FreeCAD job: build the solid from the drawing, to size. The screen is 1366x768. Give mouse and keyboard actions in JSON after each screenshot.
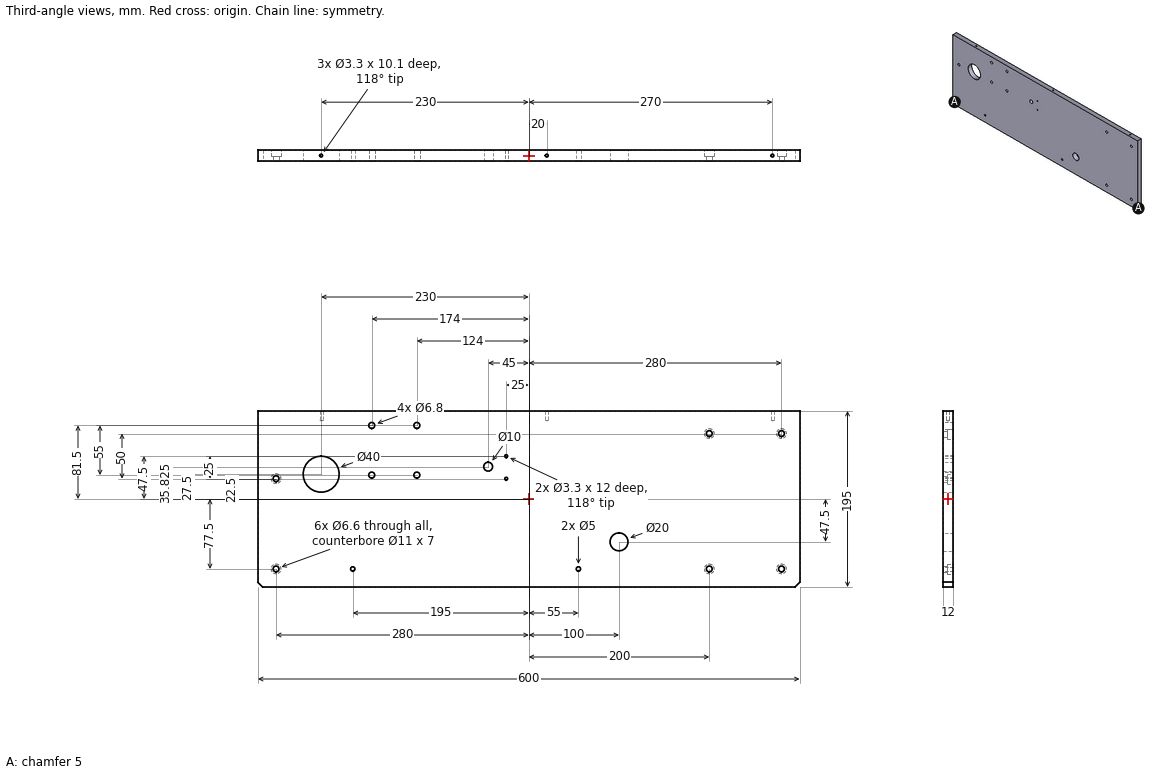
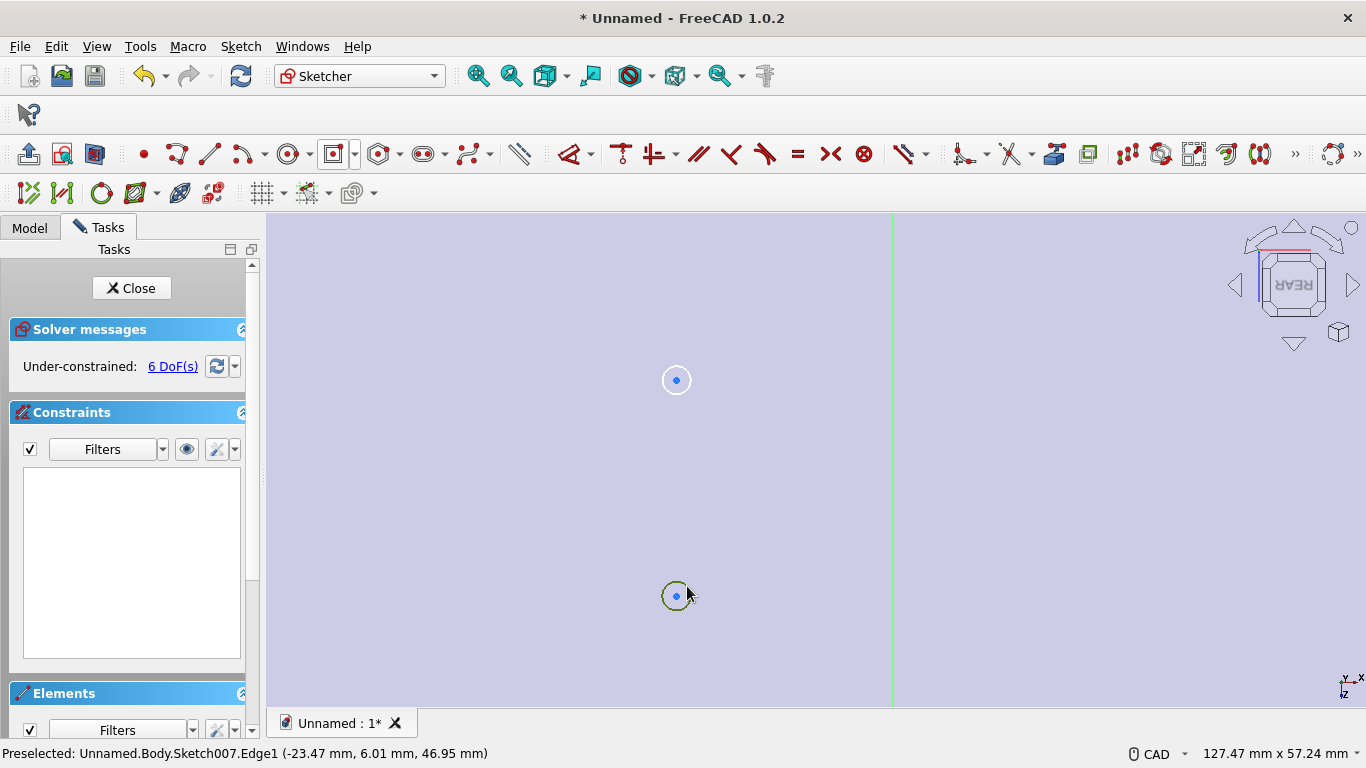
{"action": "left_click", "coordinate": [687, 370]}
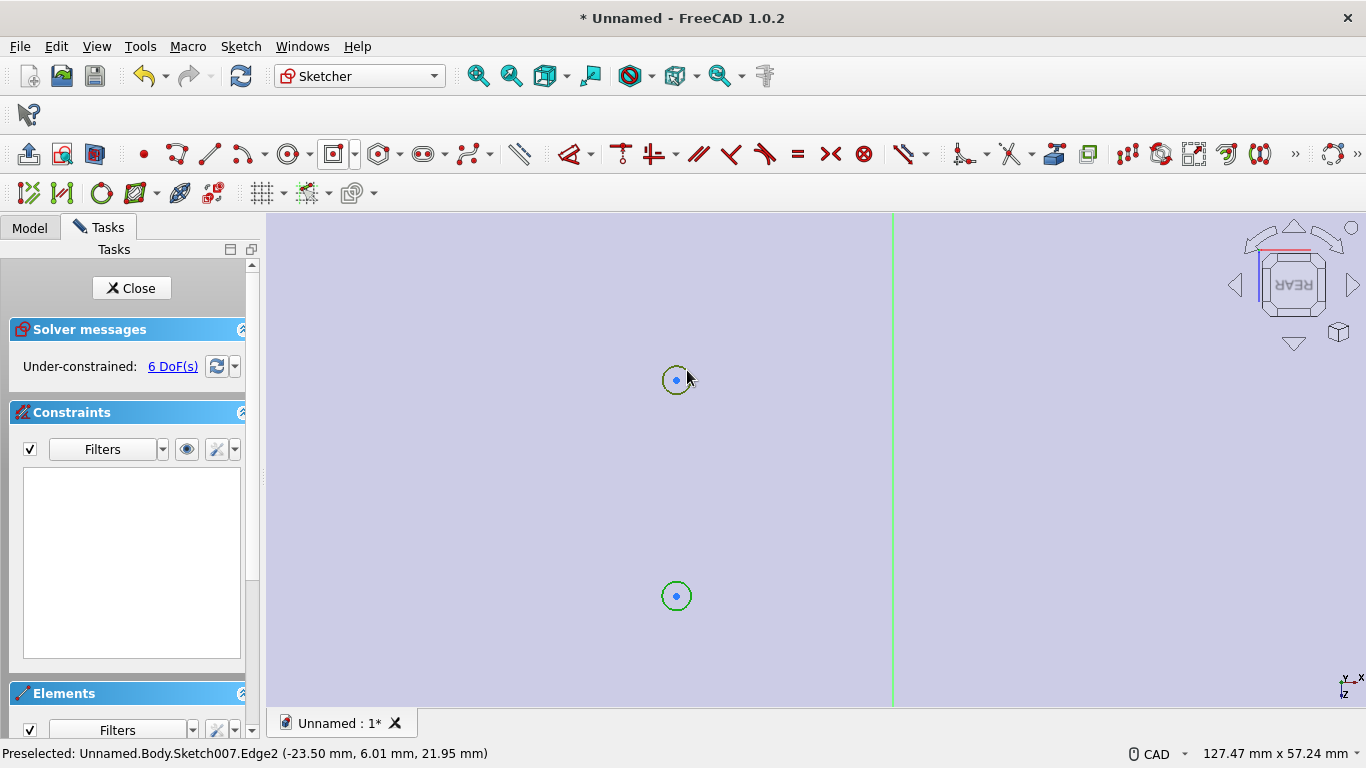
{"action": "left_click", "coordinate": [798, 154]}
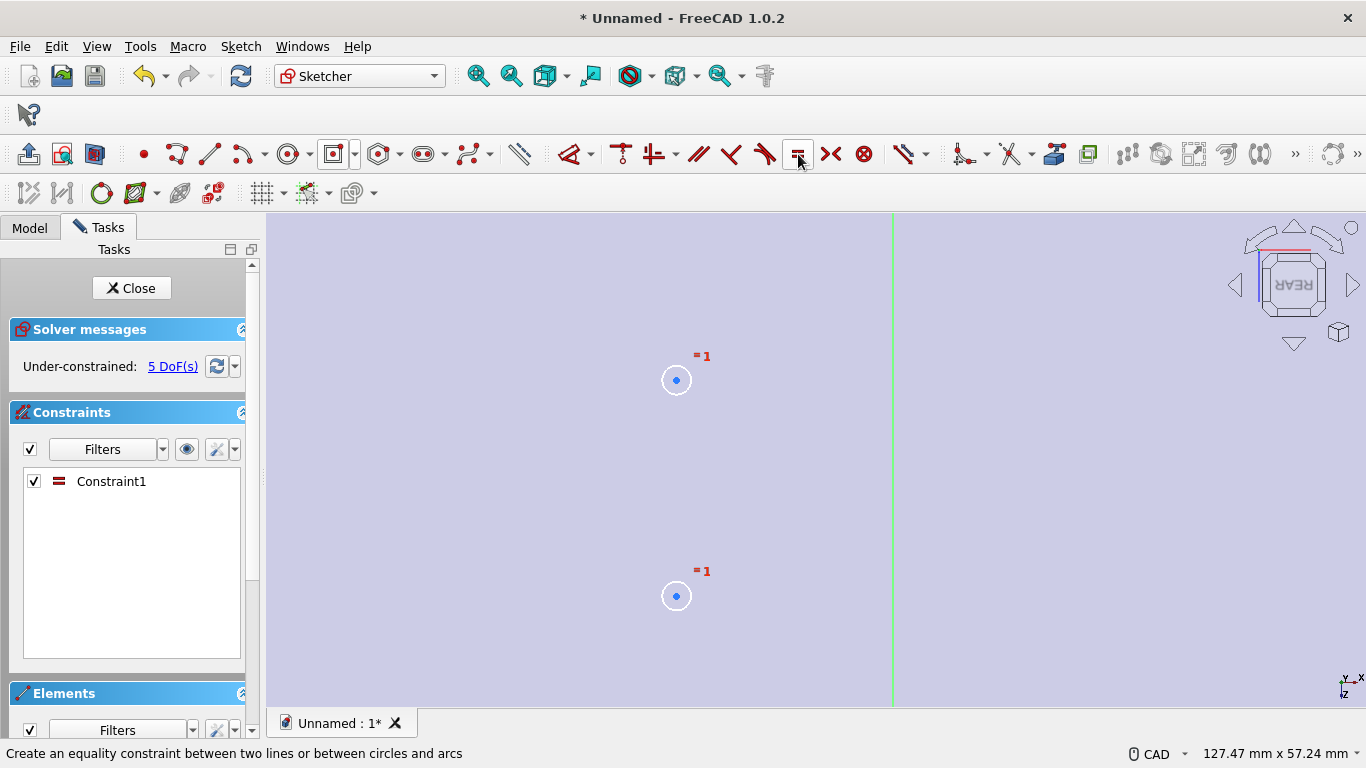
{"action": "key", "text": "d"}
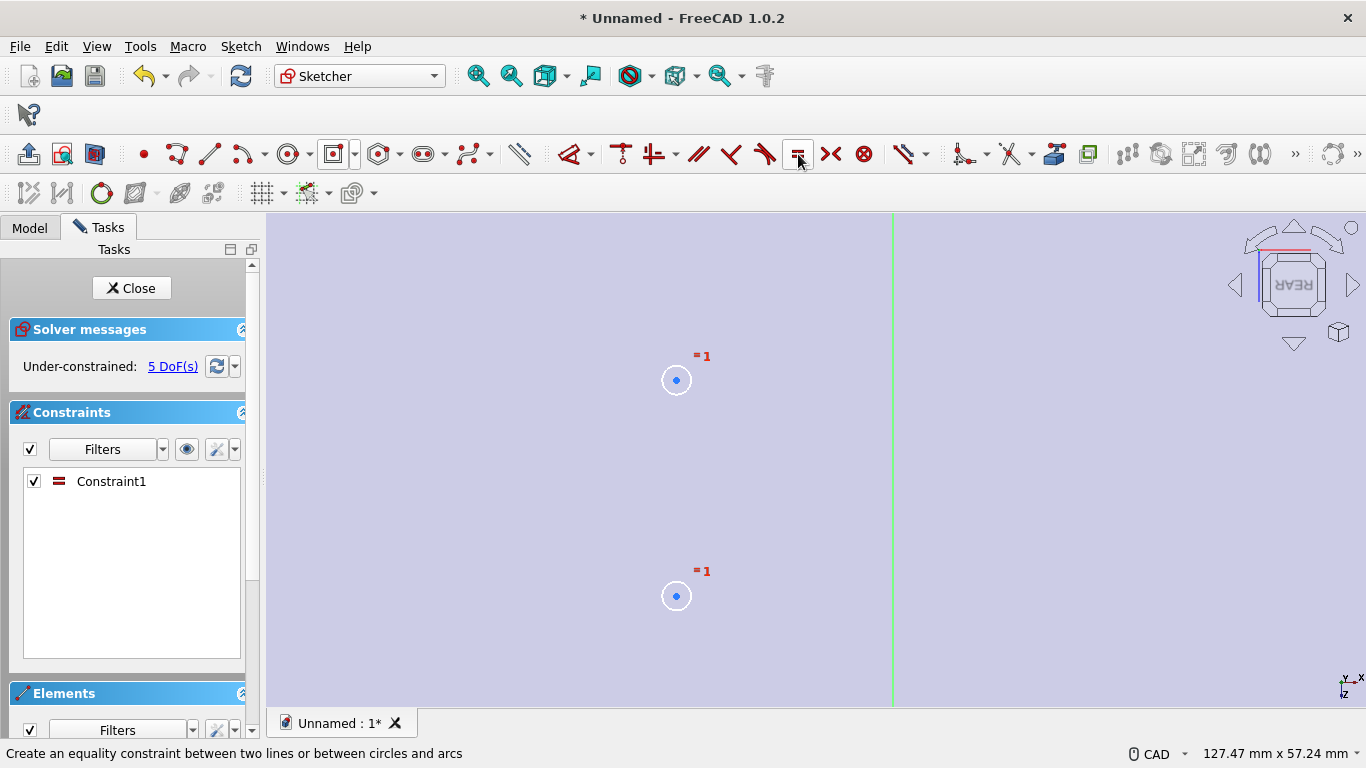
{"action": "scroll", "coordinate": [687, 586], "scroll_direction": "up", "scroll_amount": 2}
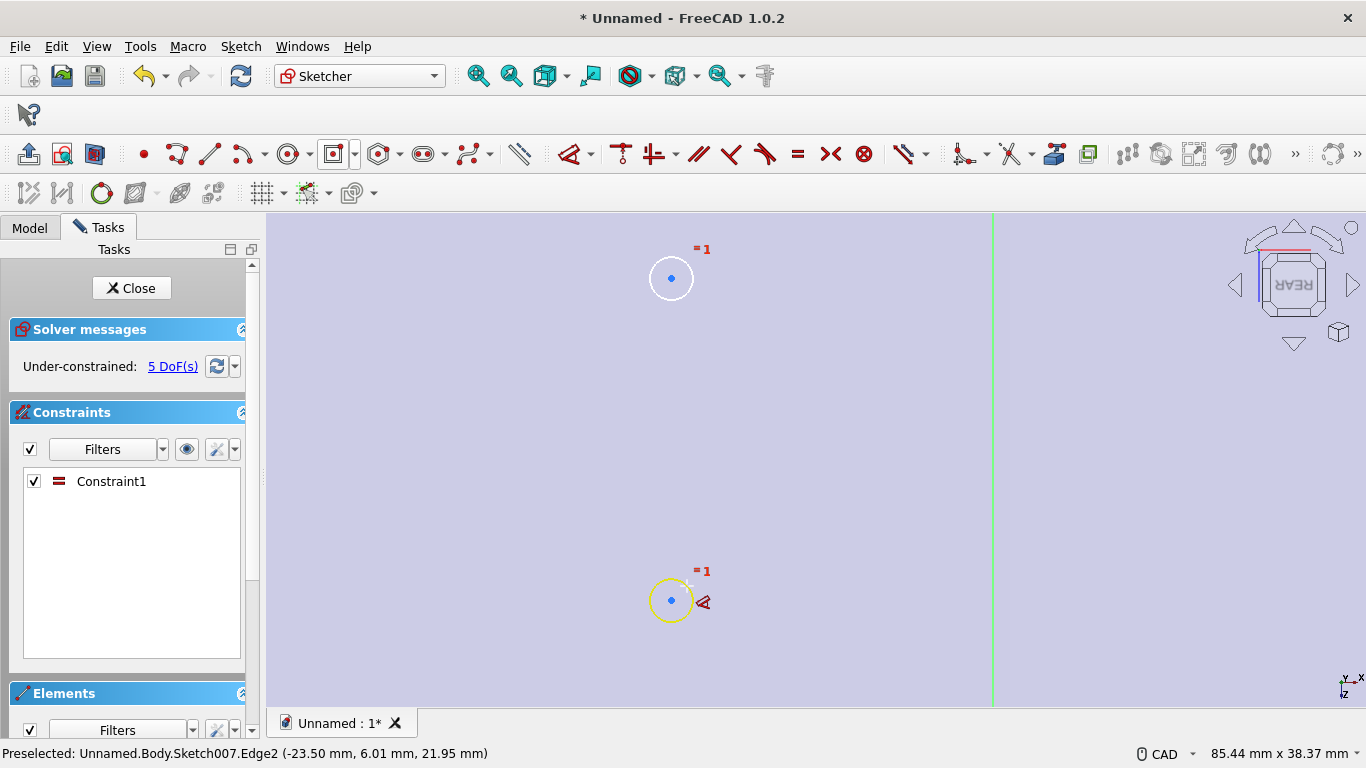
{"action": "left_click", "coordinate": [686, 585]}
{"action": "left_click", "coordinate": [708, 562]}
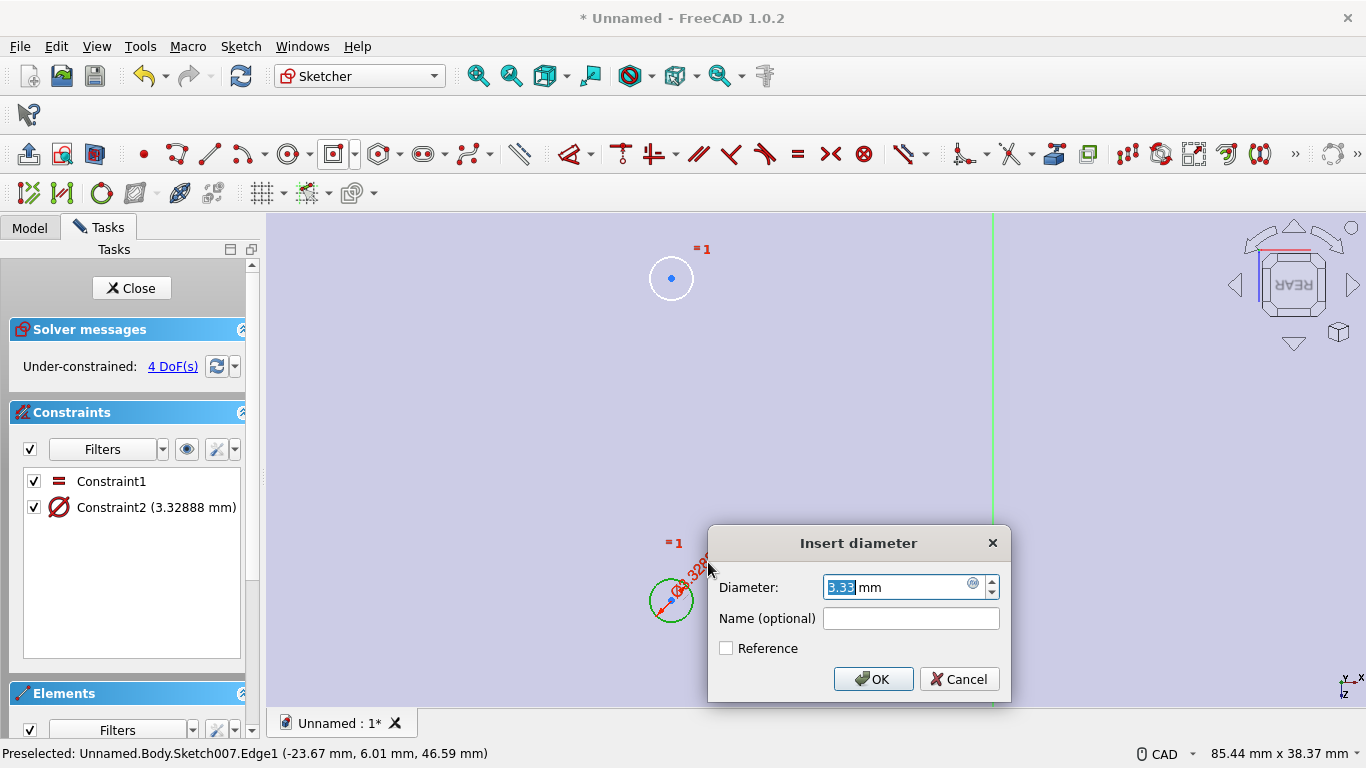
{"action": "type", "text": "3.3"}
{"action": "key", "text": "Return"}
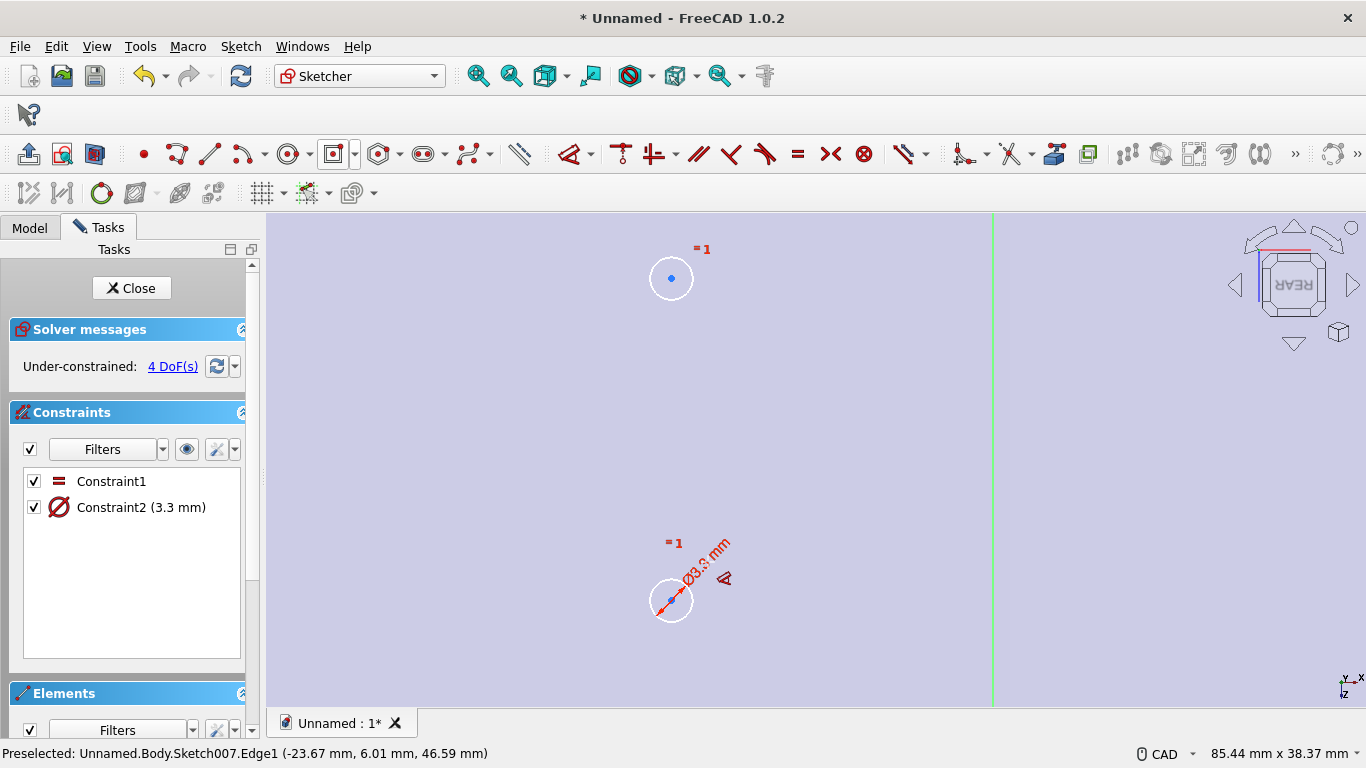
{"action": "left_click", "coordinate": [671, 601]}
{"action": "left_click", "coordinate": [832, 635]}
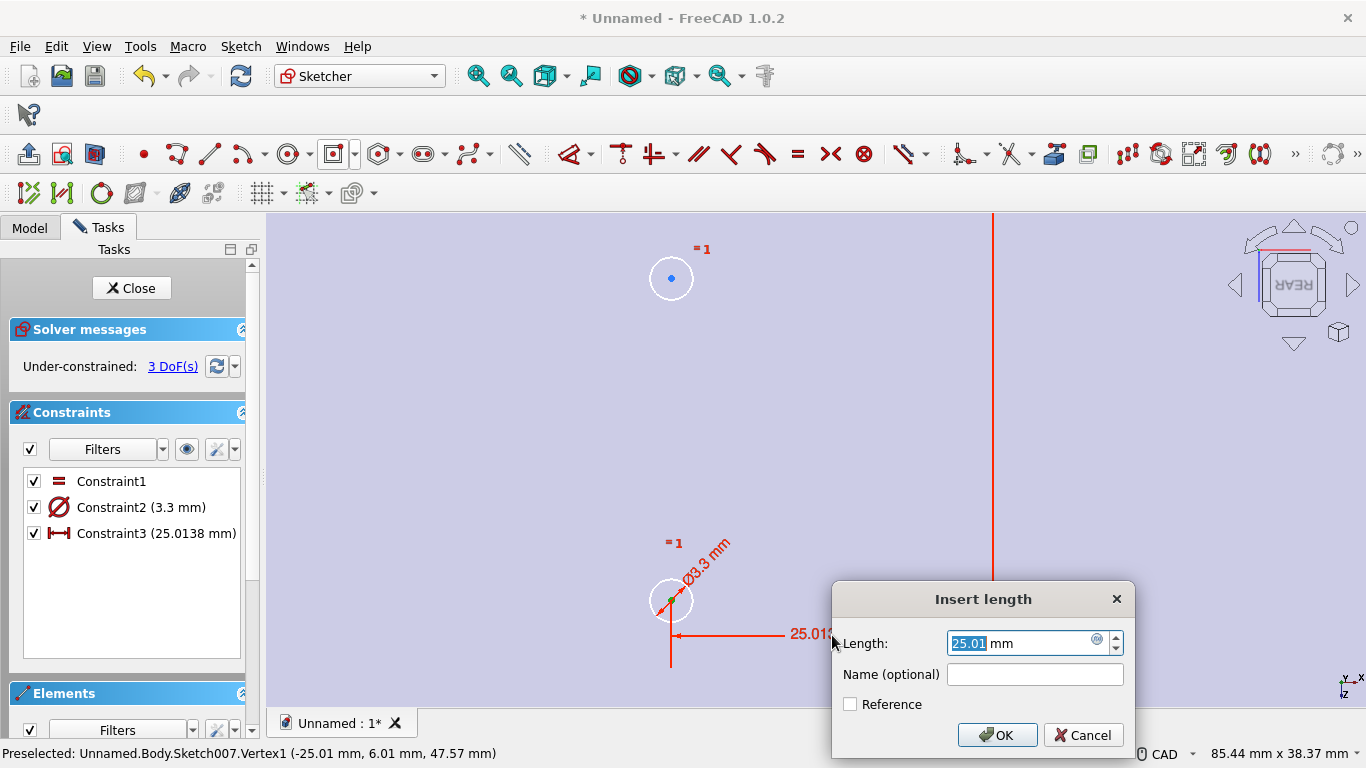
{"action": "type", "text": "25"}
{"action": "key", "text": "Return"}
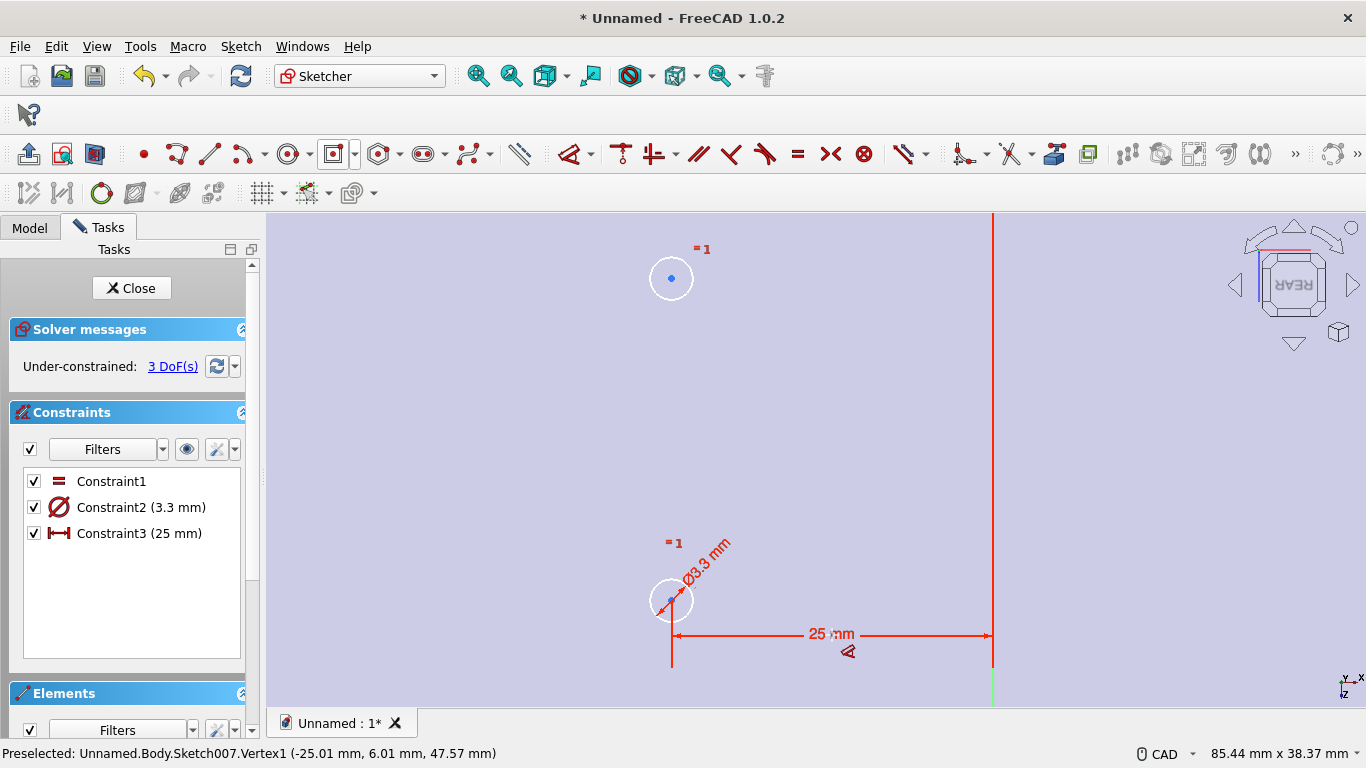
{"action": "left_click", "coordinate": [671, 279]}
{"action": "left_click", "coordinate": [832, 313]}